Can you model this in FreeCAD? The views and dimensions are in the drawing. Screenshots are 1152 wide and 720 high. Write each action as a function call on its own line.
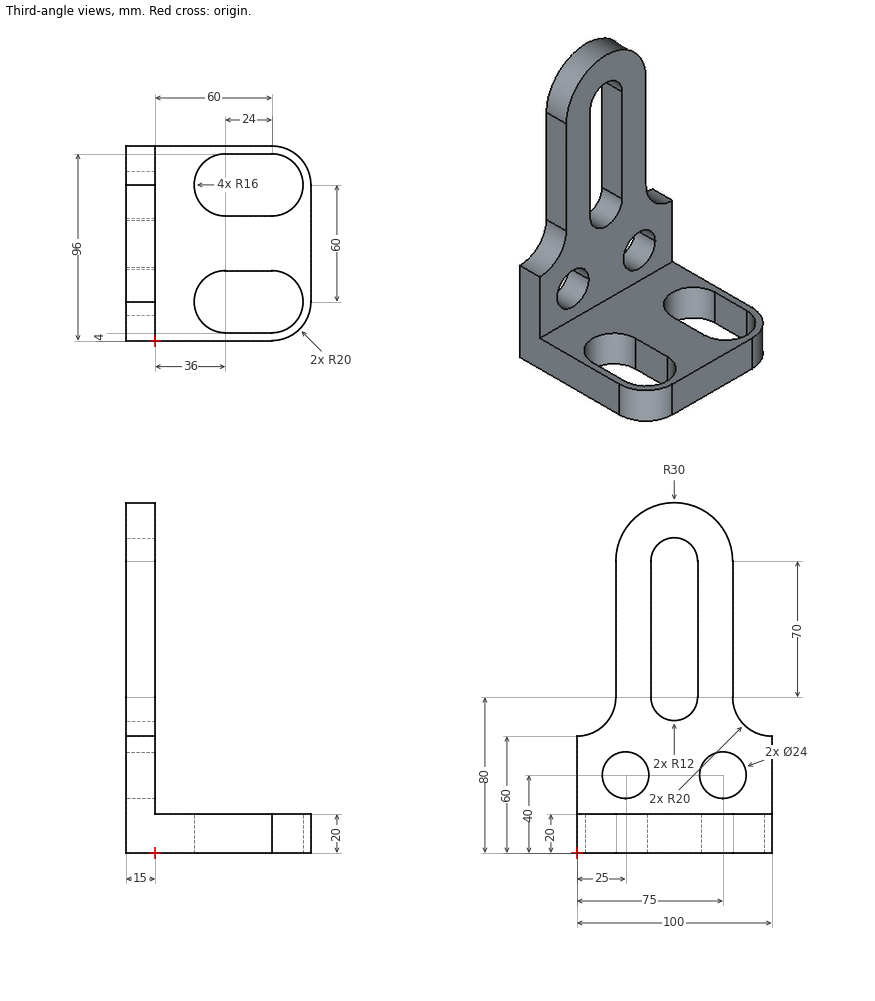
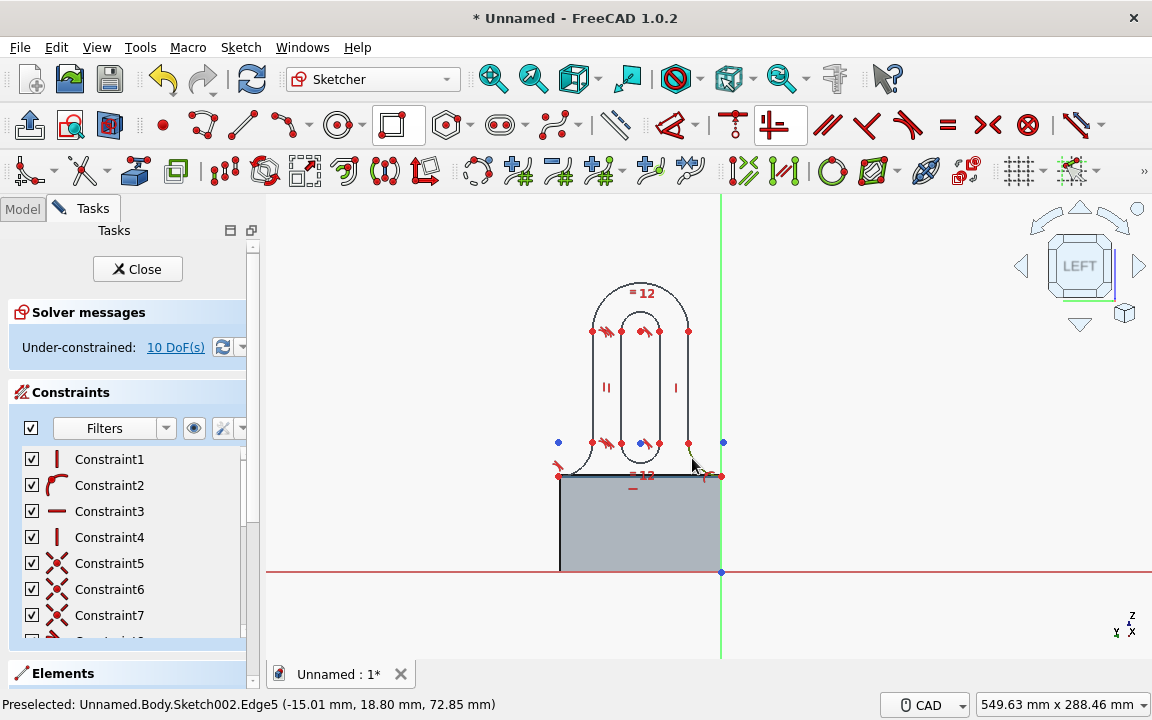
click(908, 126)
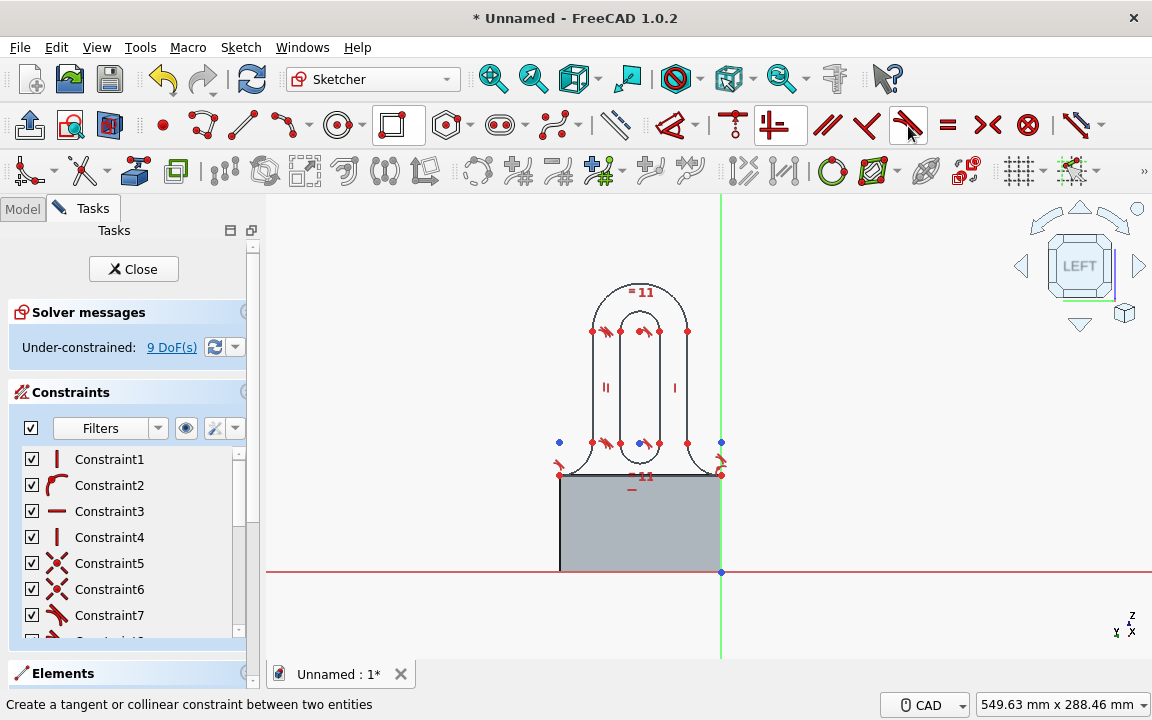
click(687, 410)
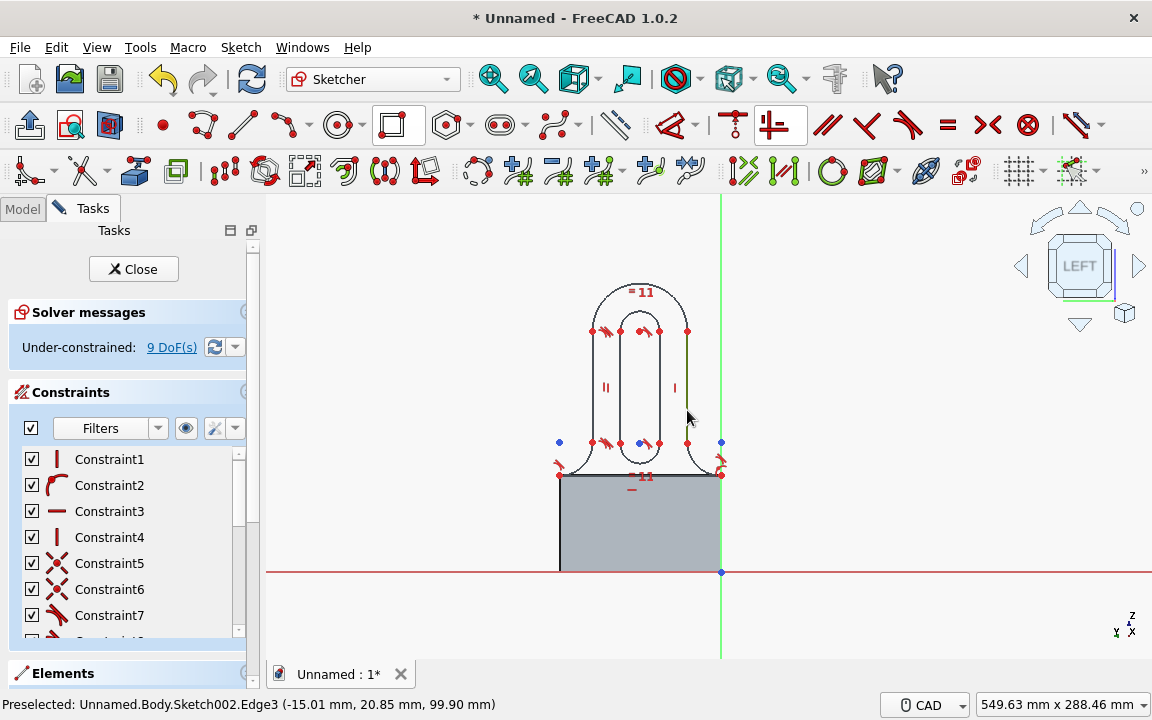
click(692, 458)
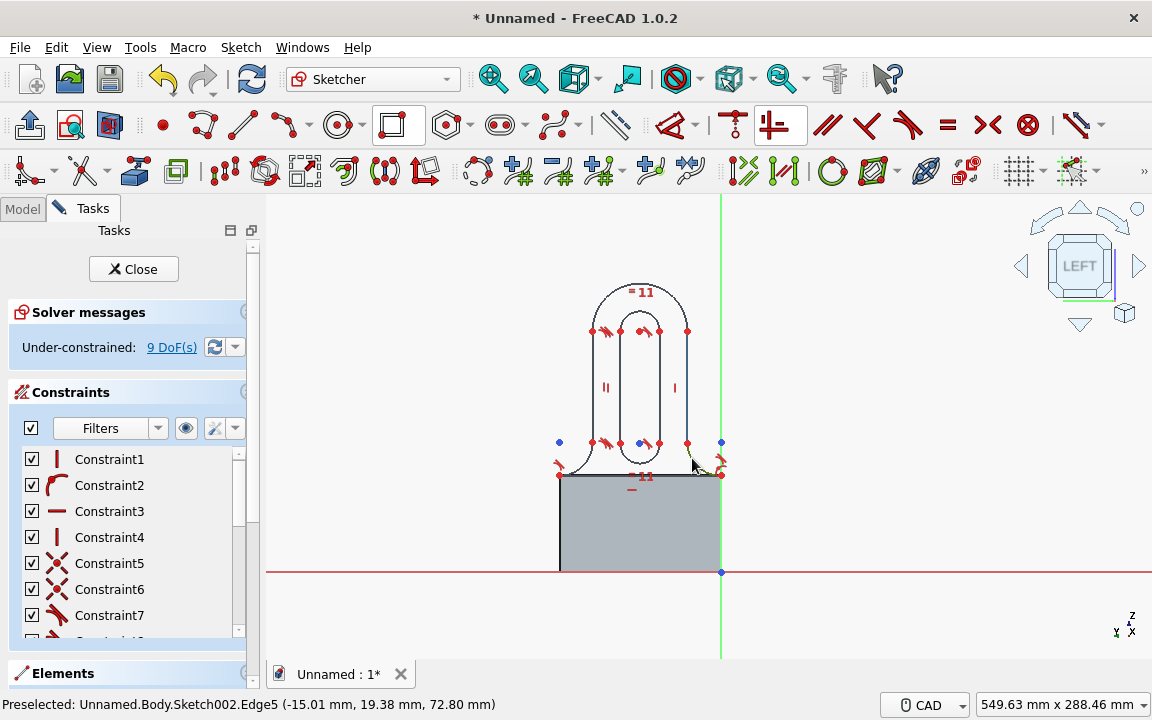
click(908, 126)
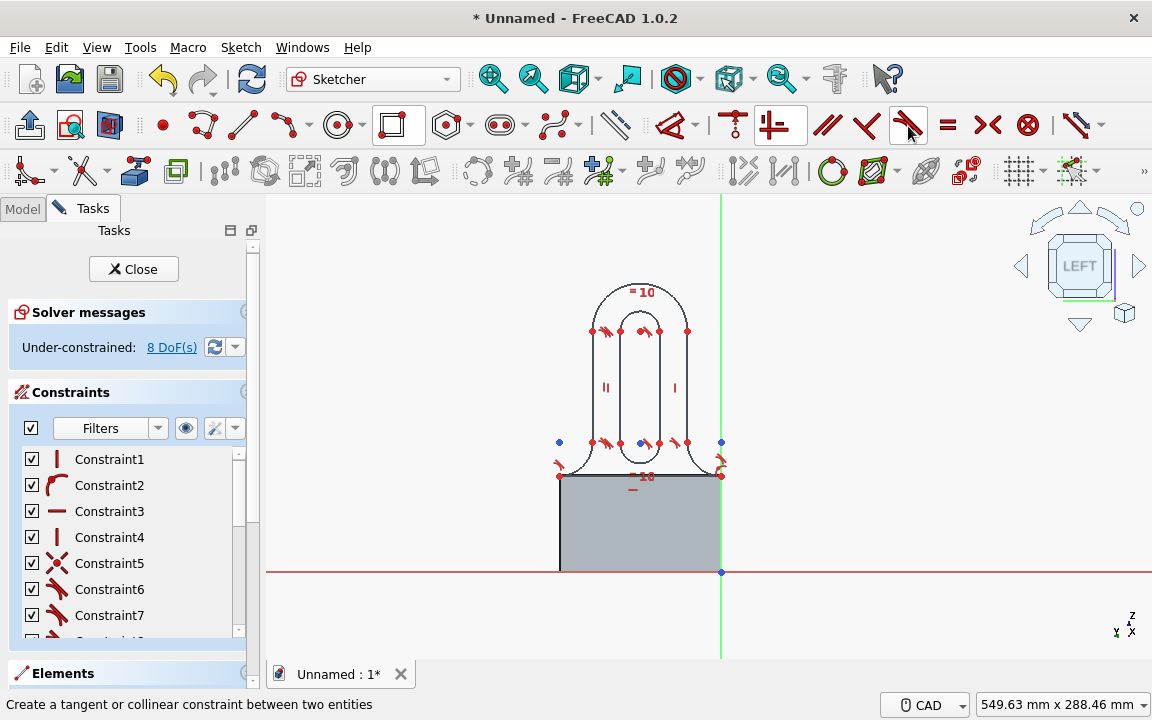
click(687, 409)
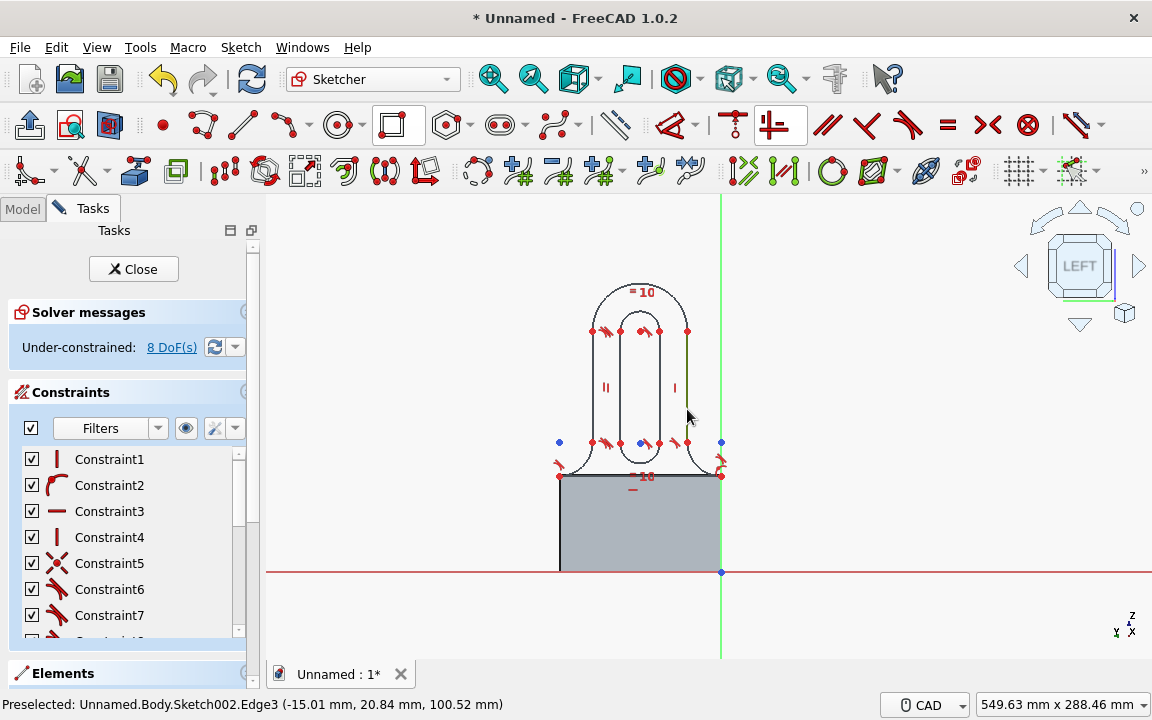
click(668, 293)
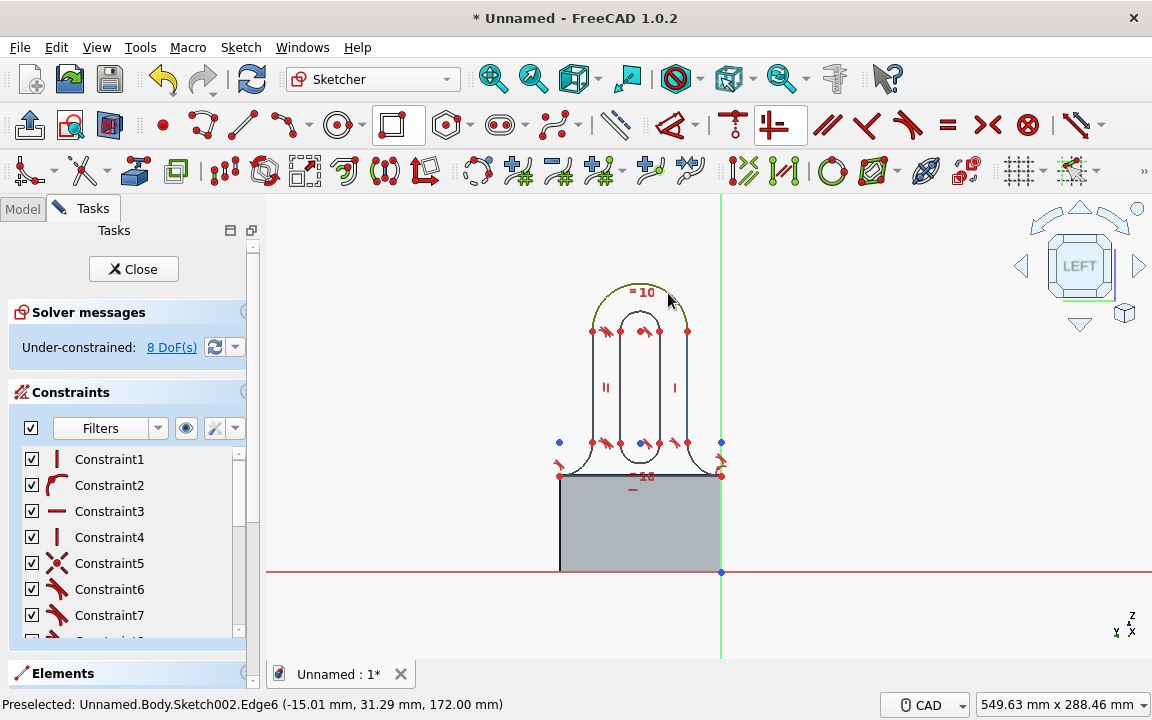
click(908, 126)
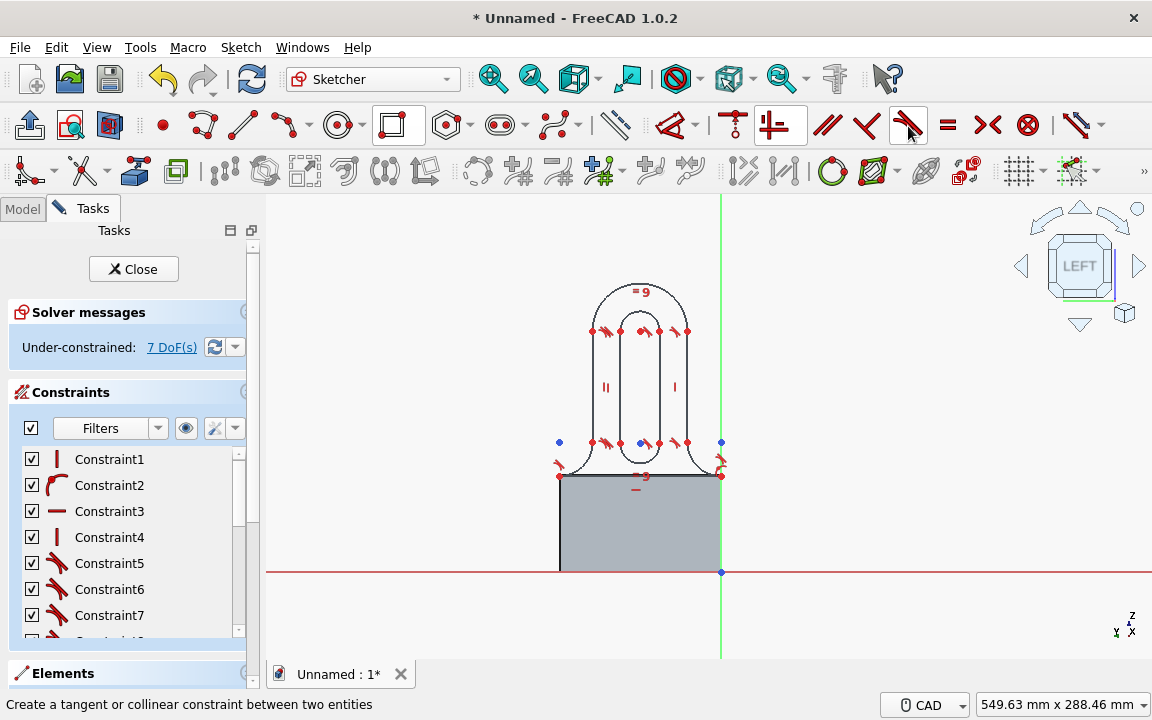
click(589, 458)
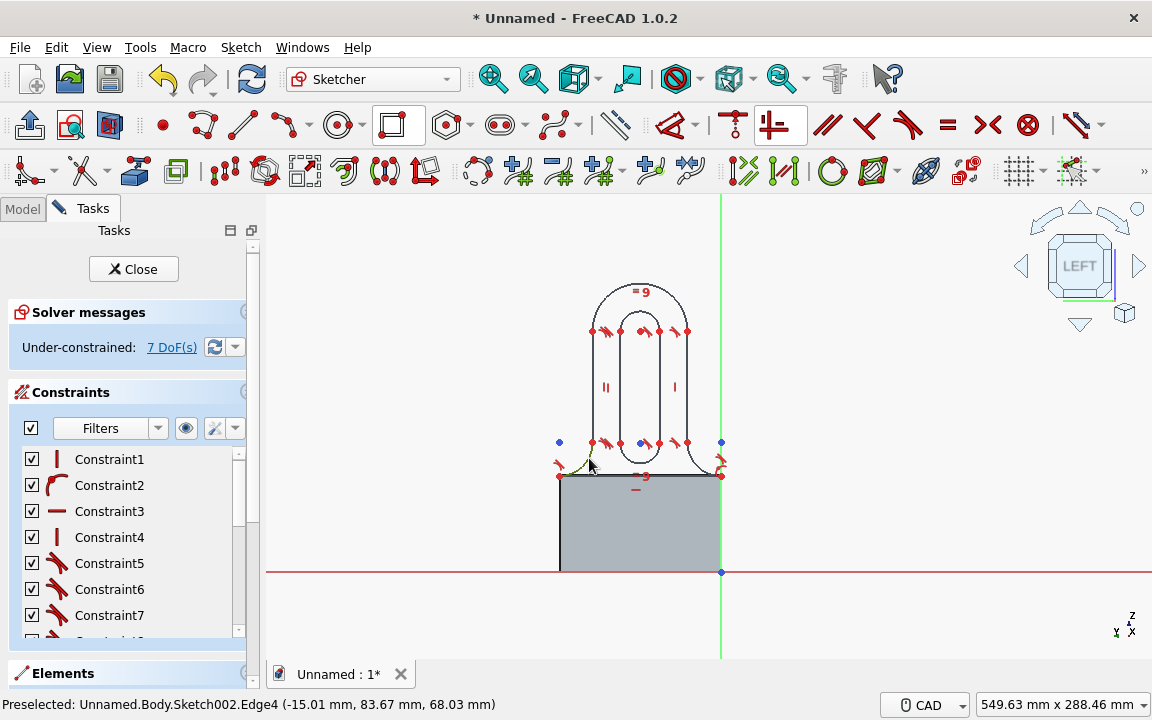
click(691, 458)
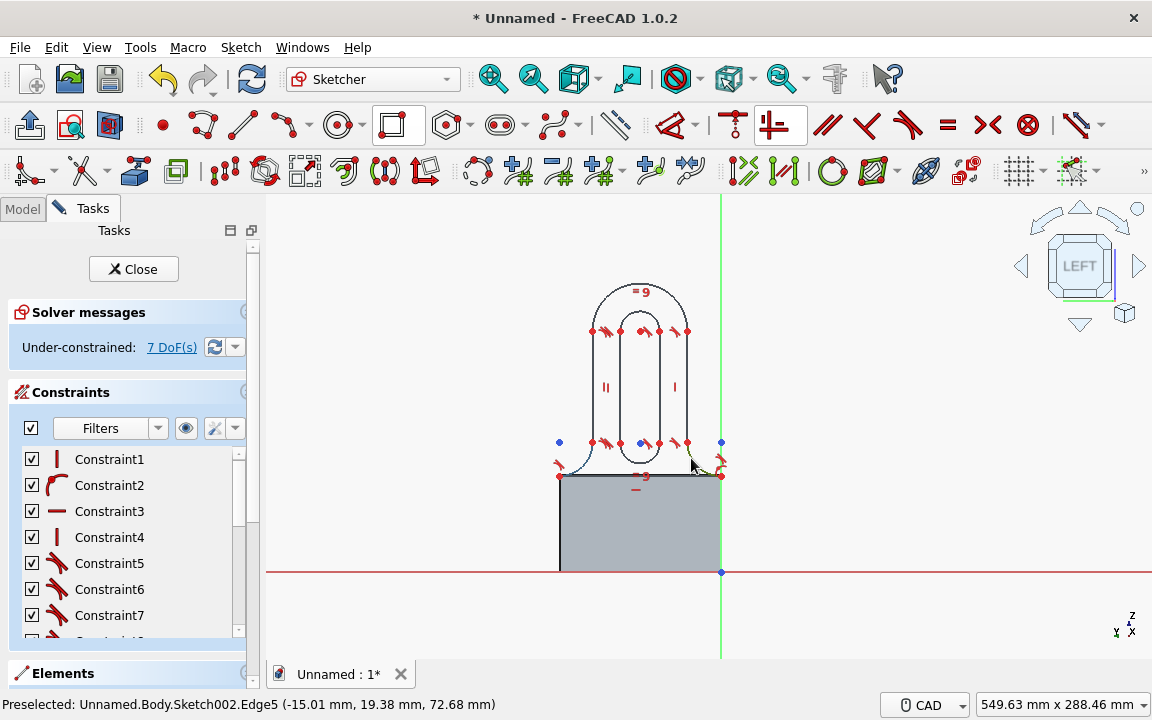
click(948, 126)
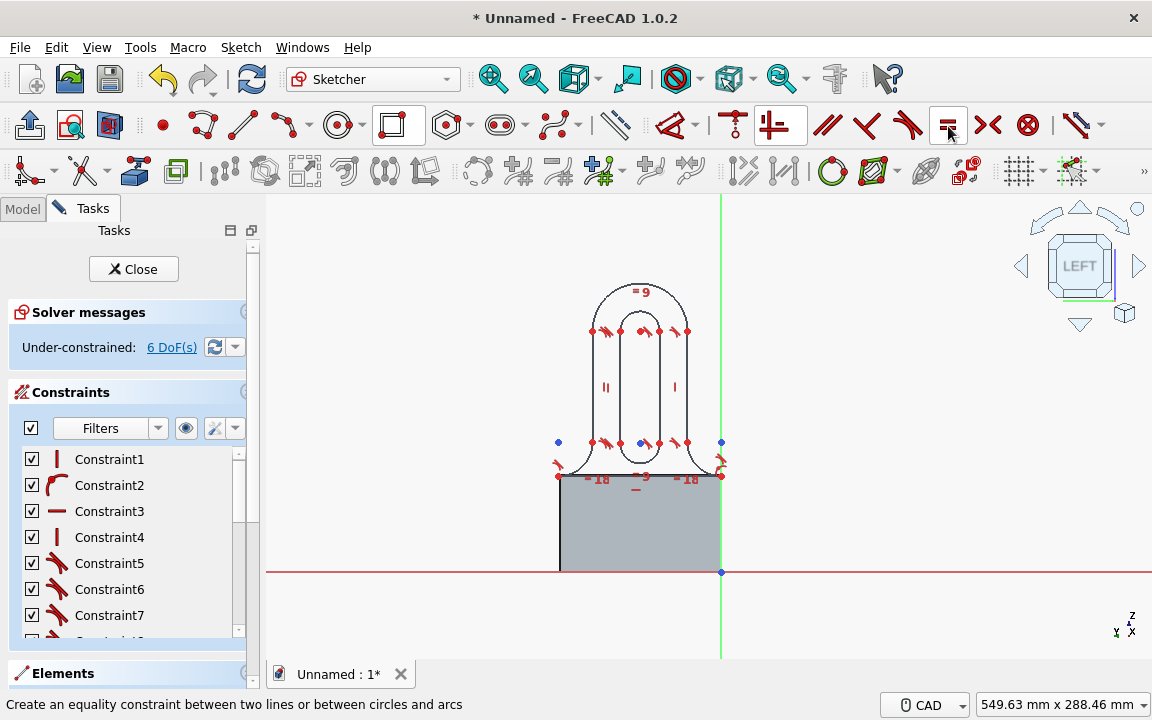
click(670, 126)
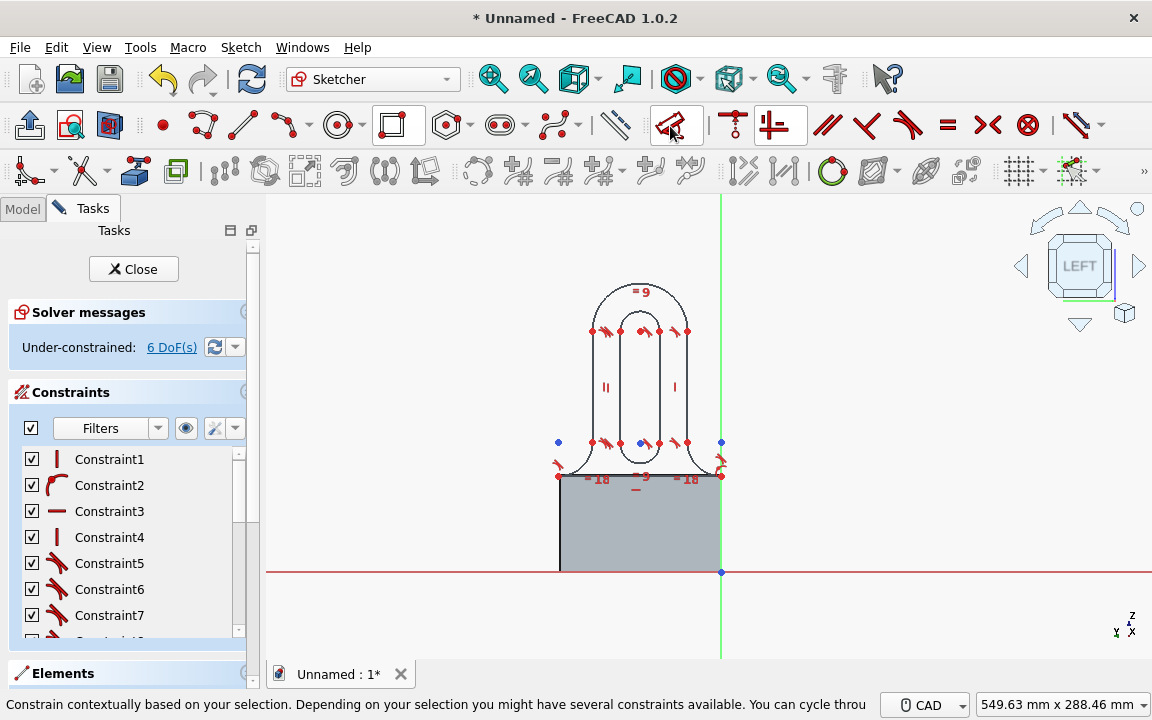
scroll(589, 458, up, 2)